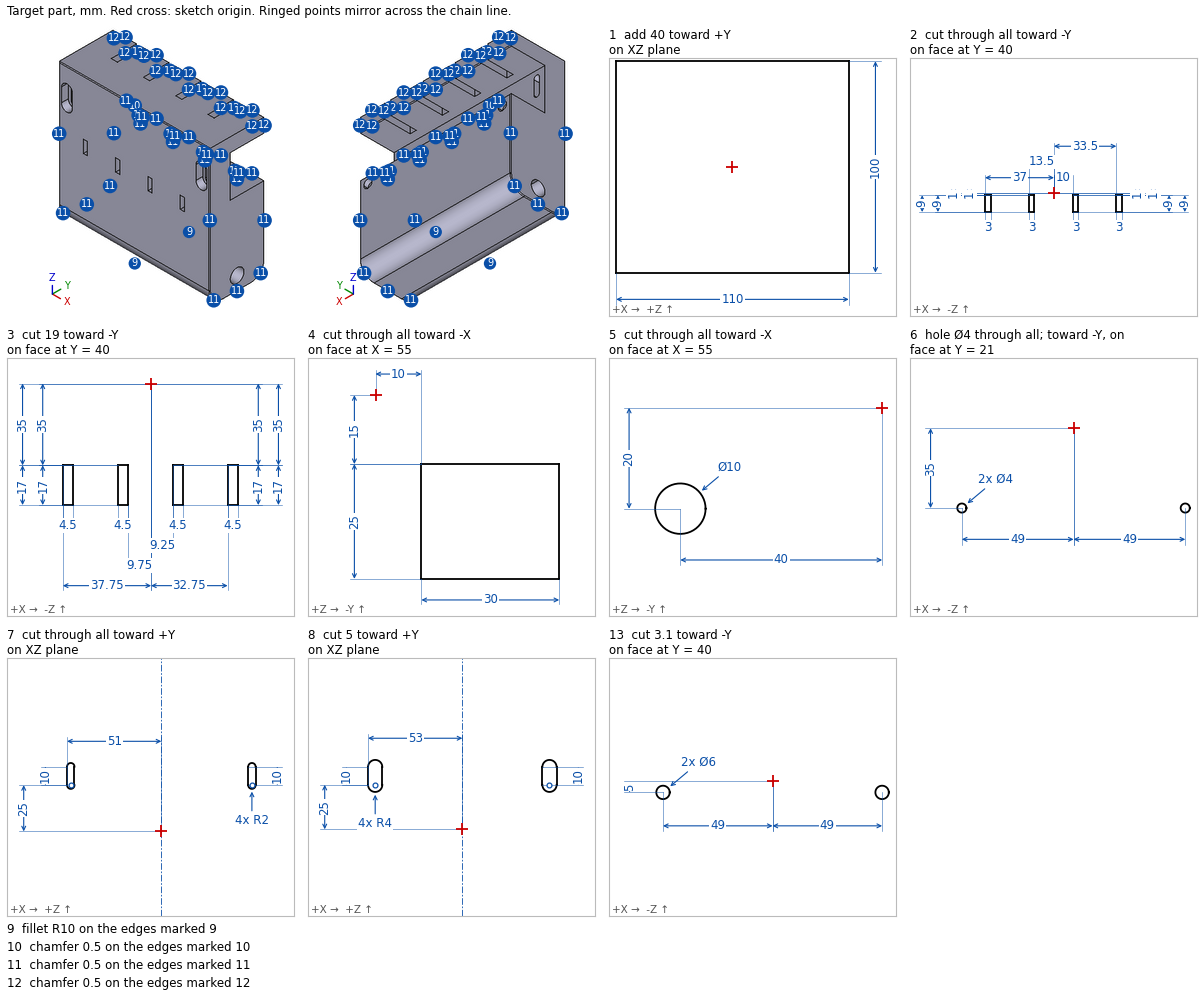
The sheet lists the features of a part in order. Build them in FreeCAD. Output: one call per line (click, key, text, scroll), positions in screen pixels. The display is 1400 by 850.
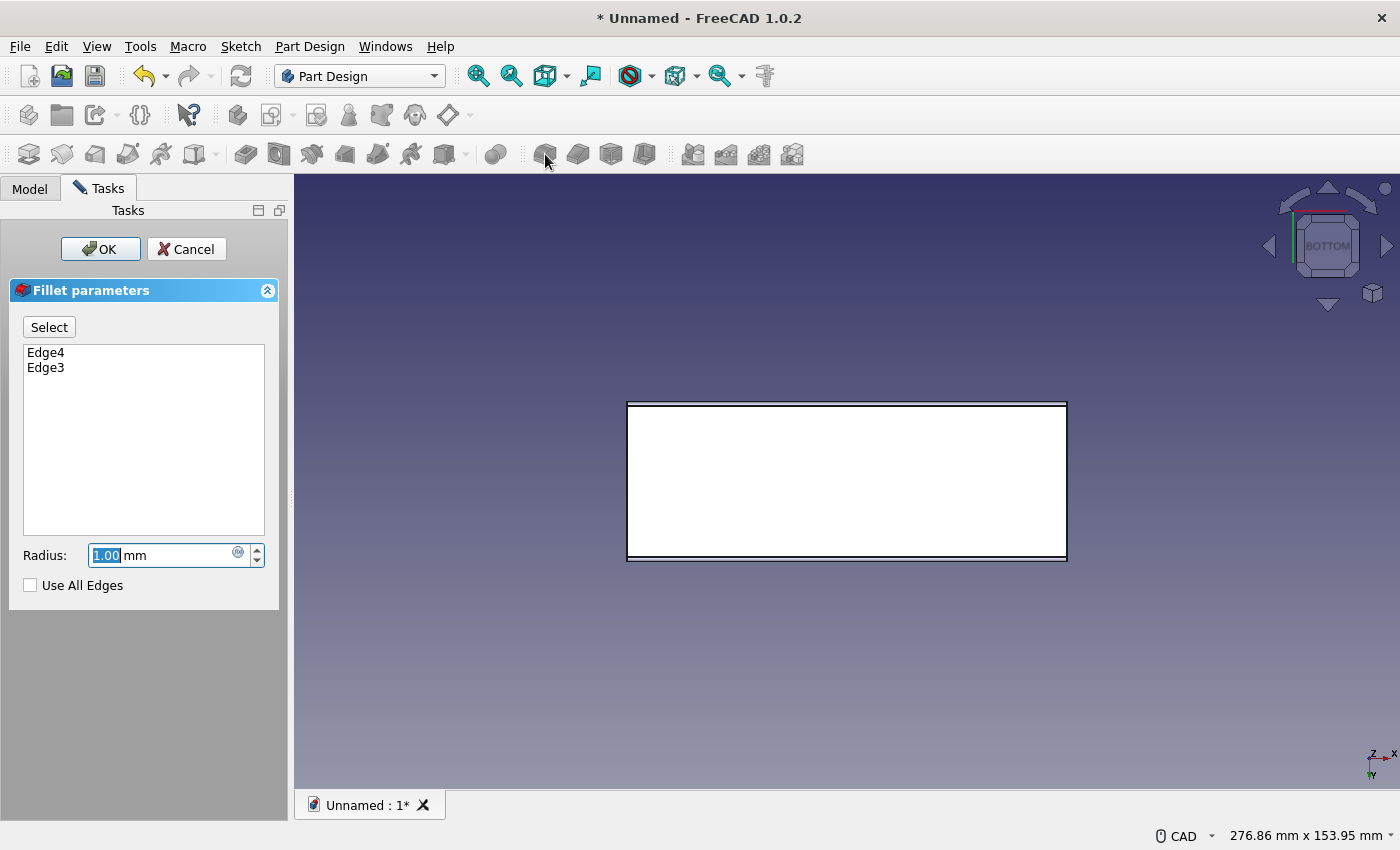
text(10)
key(Tab)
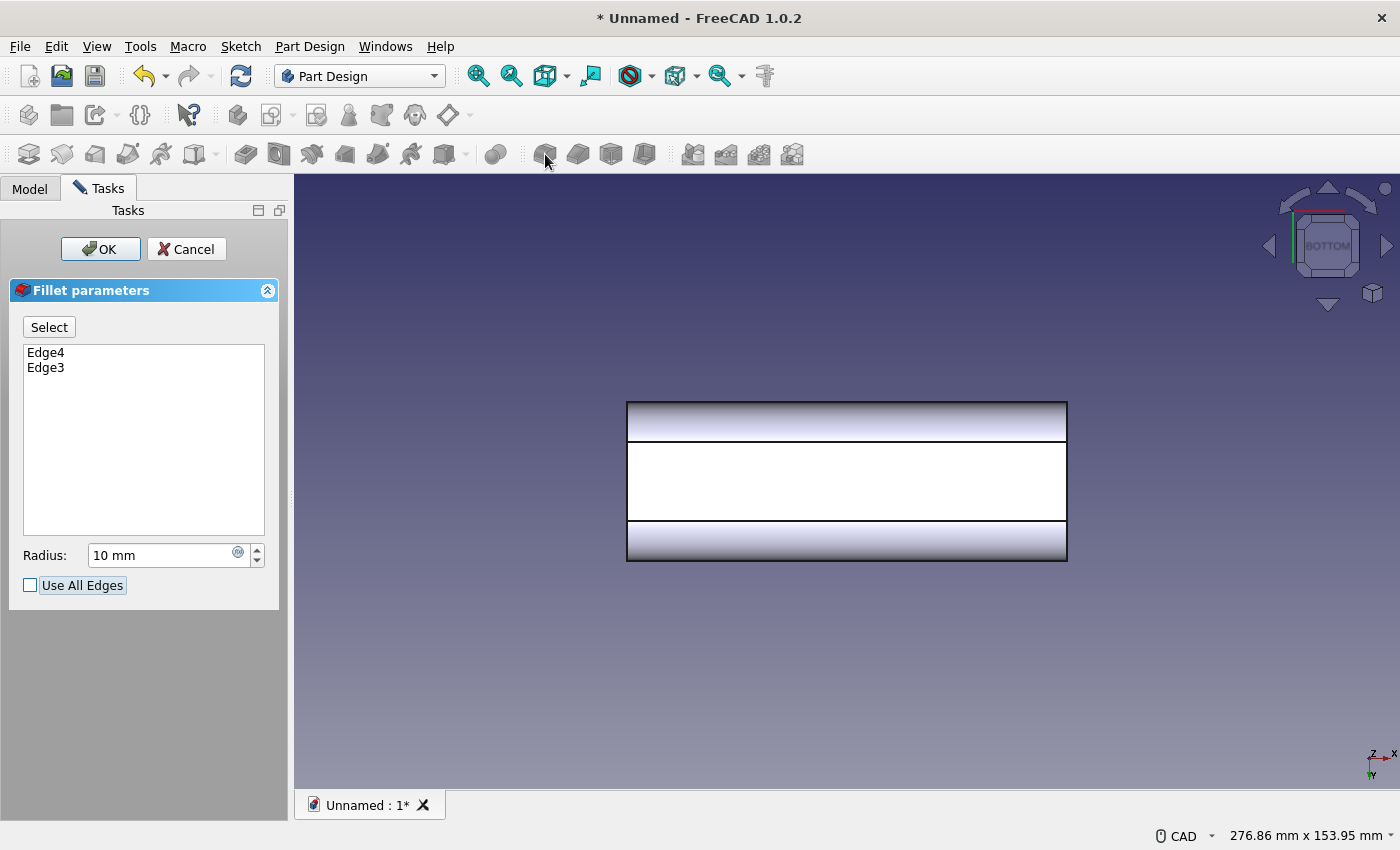
click(101, 249)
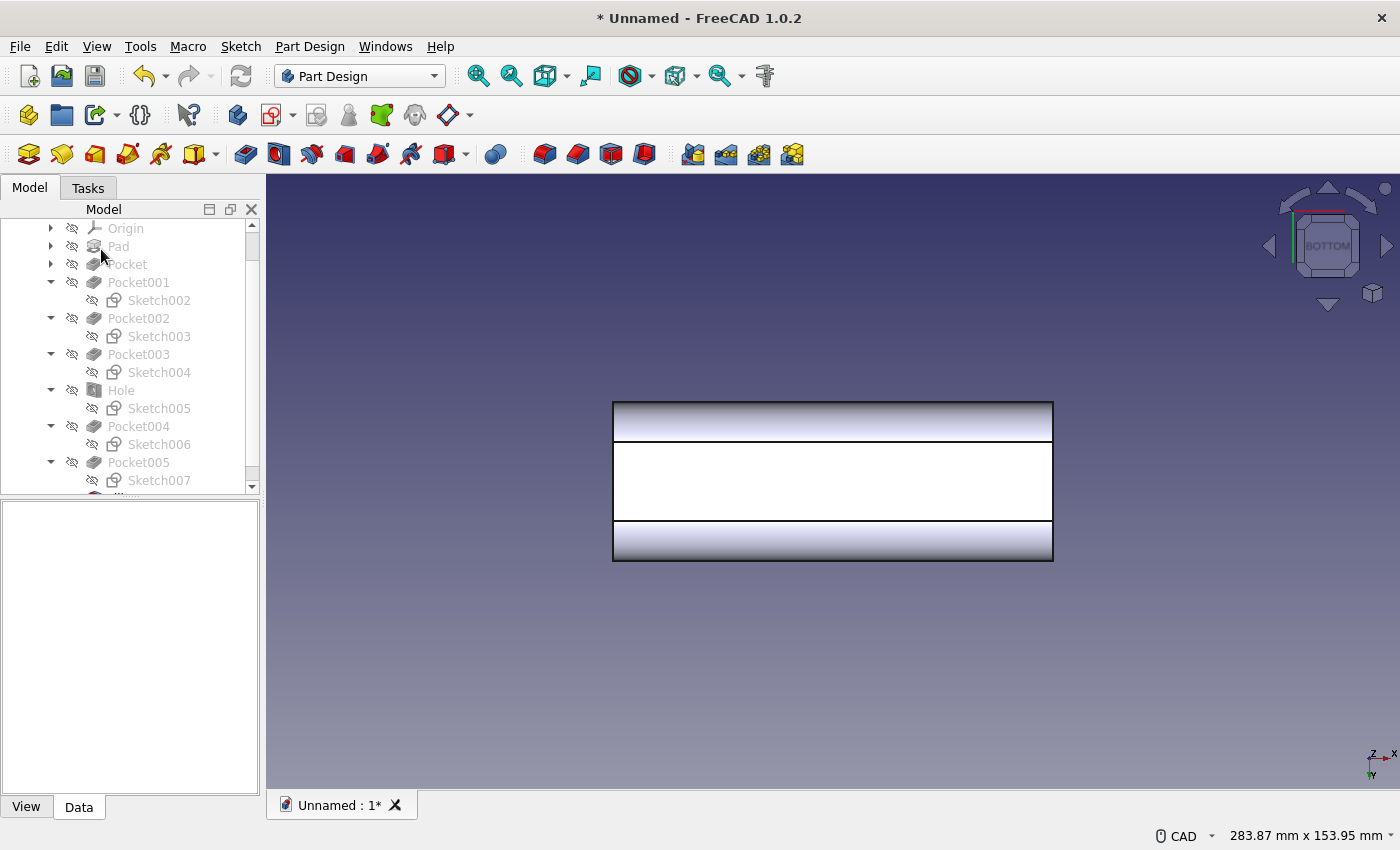
key(v)
key(f)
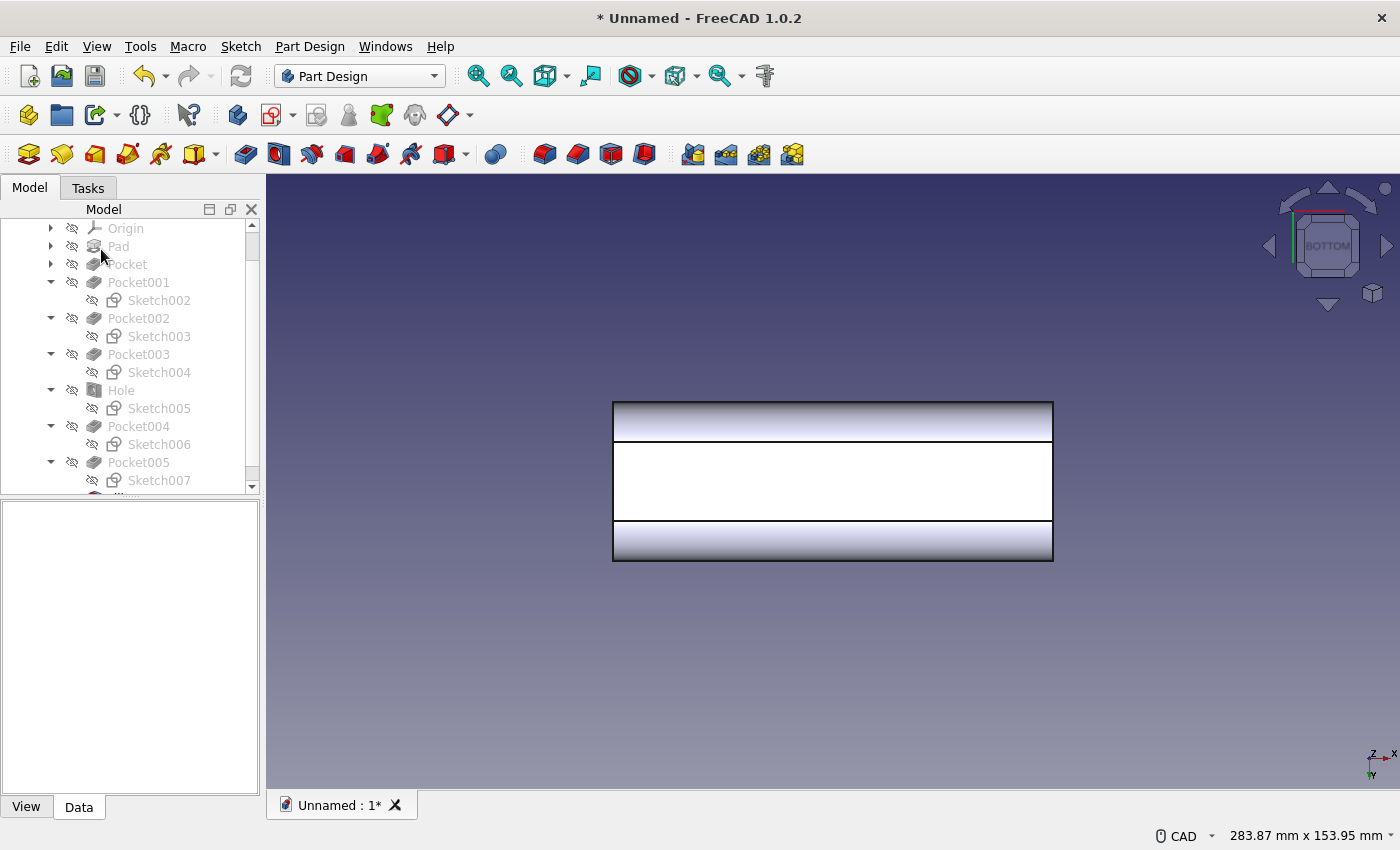
key(0)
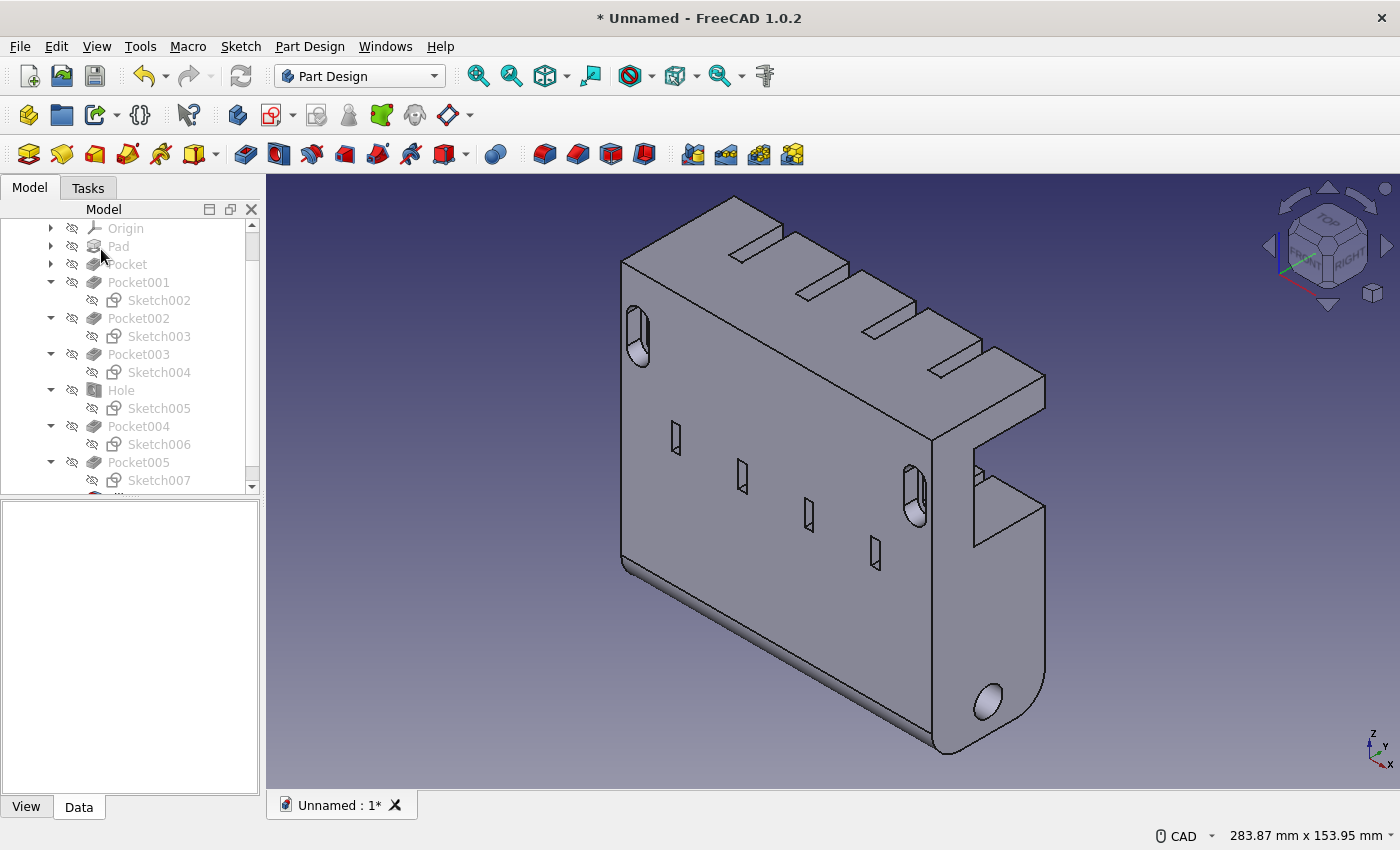
click(777, 350)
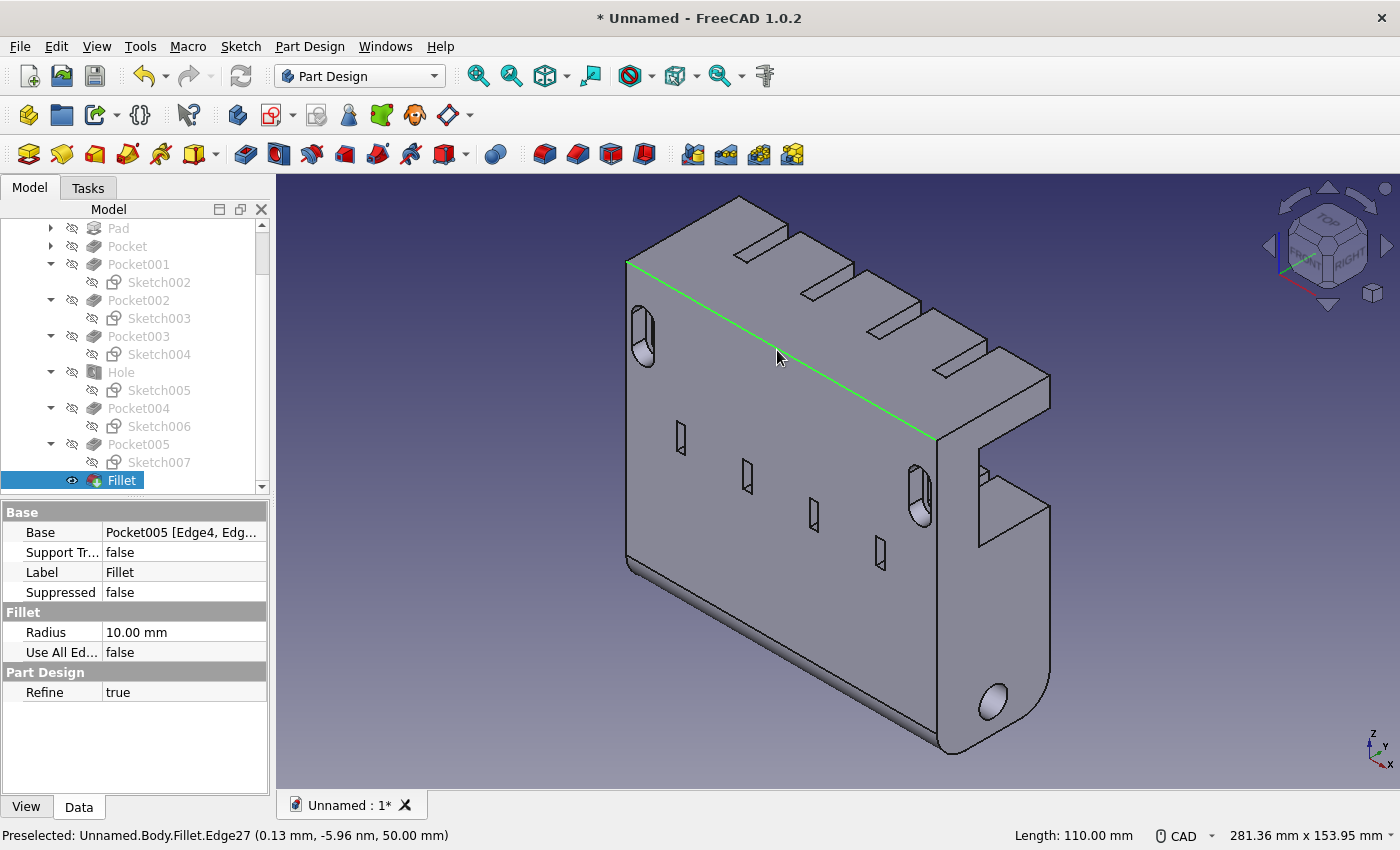
click(578, 154)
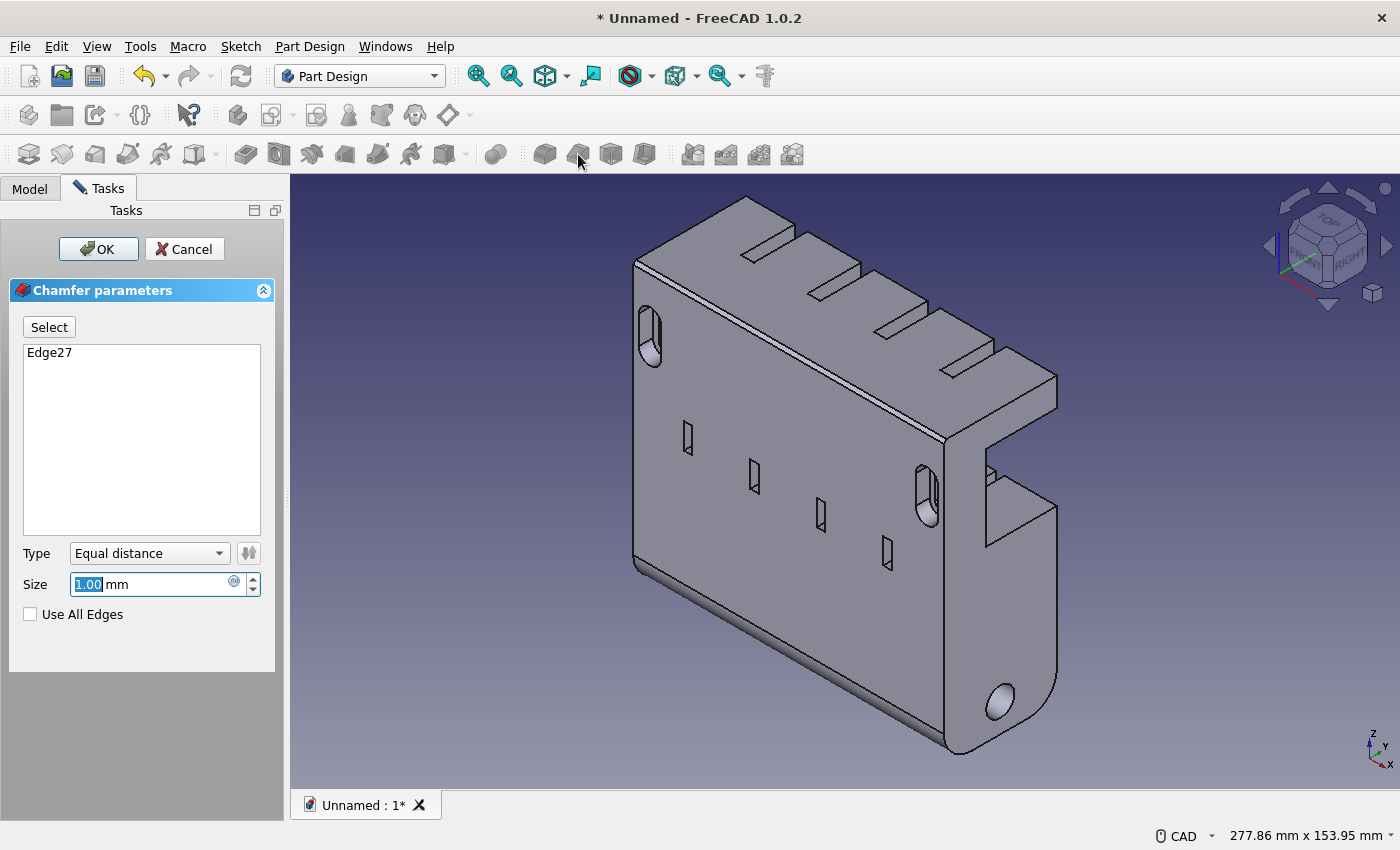
text(0.5)
key(Tab)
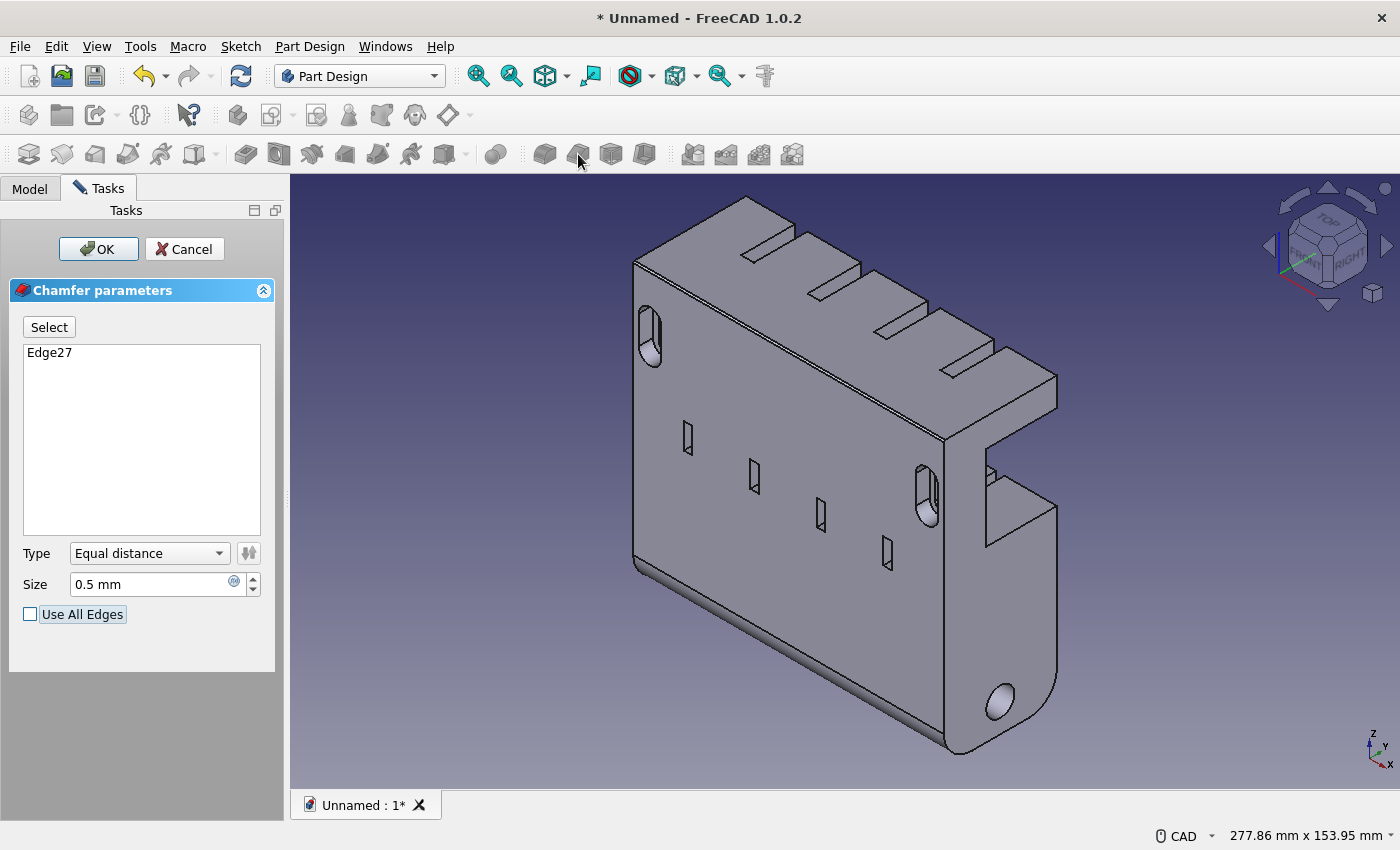
click(99, 249)